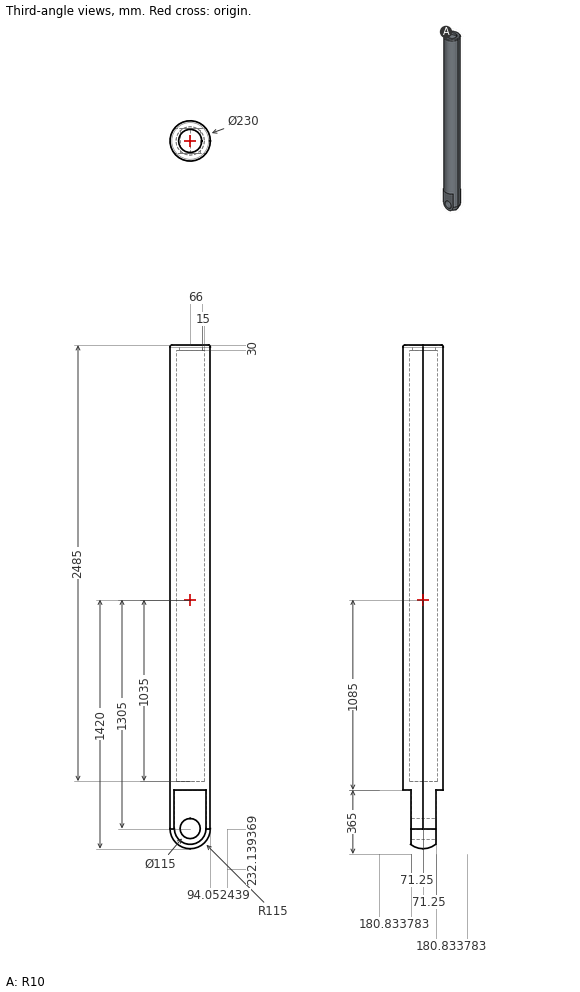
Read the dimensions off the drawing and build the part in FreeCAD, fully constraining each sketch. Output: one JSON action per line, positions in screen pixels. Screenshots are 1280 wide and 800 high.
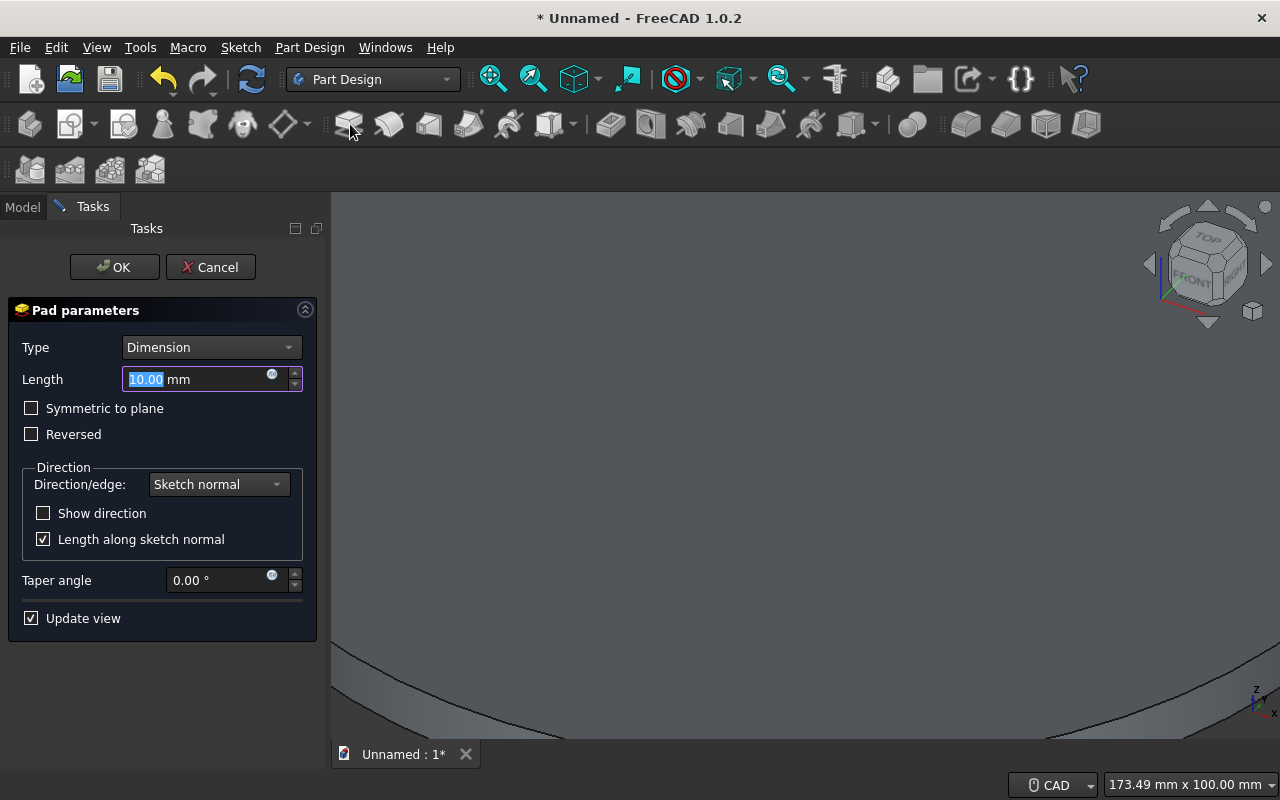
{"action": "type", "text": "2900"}
{"action": "key", "text": "Tab"}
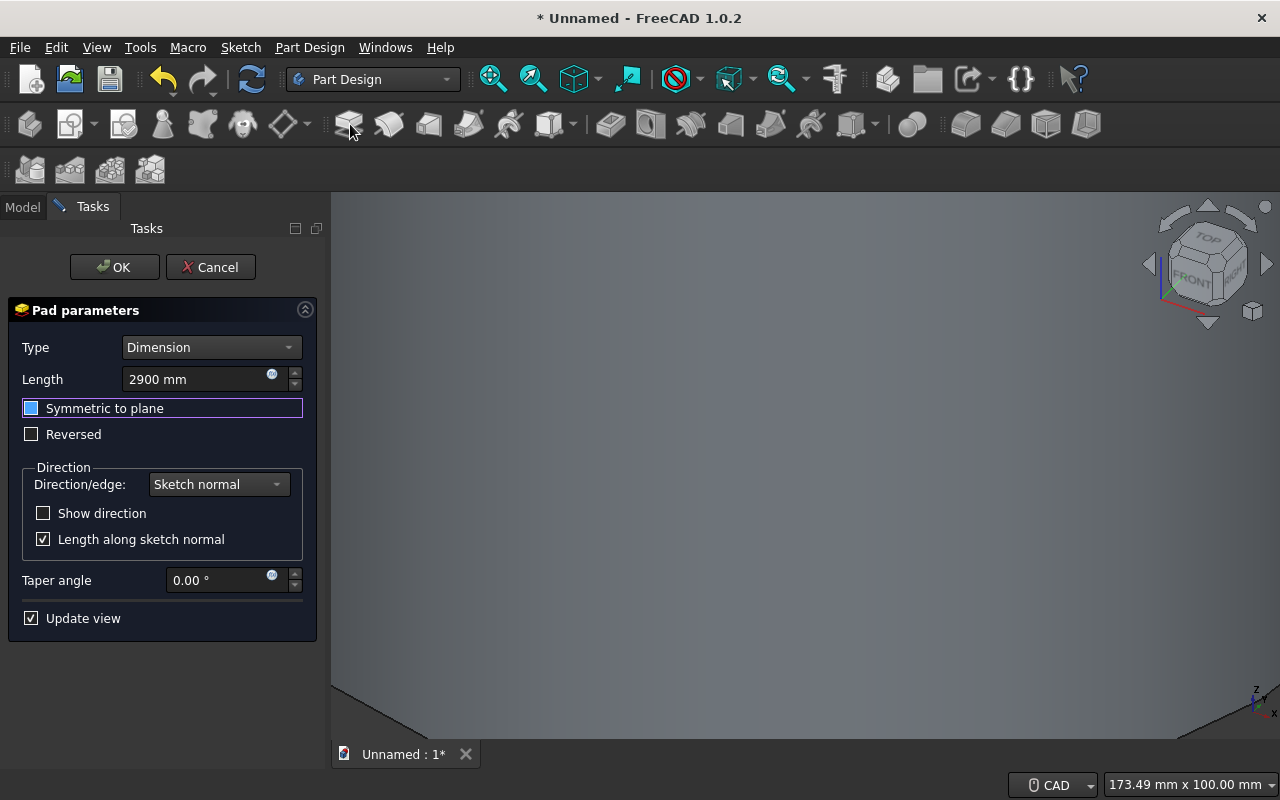
{"action": "left_click", "coordinate": [30, 408]}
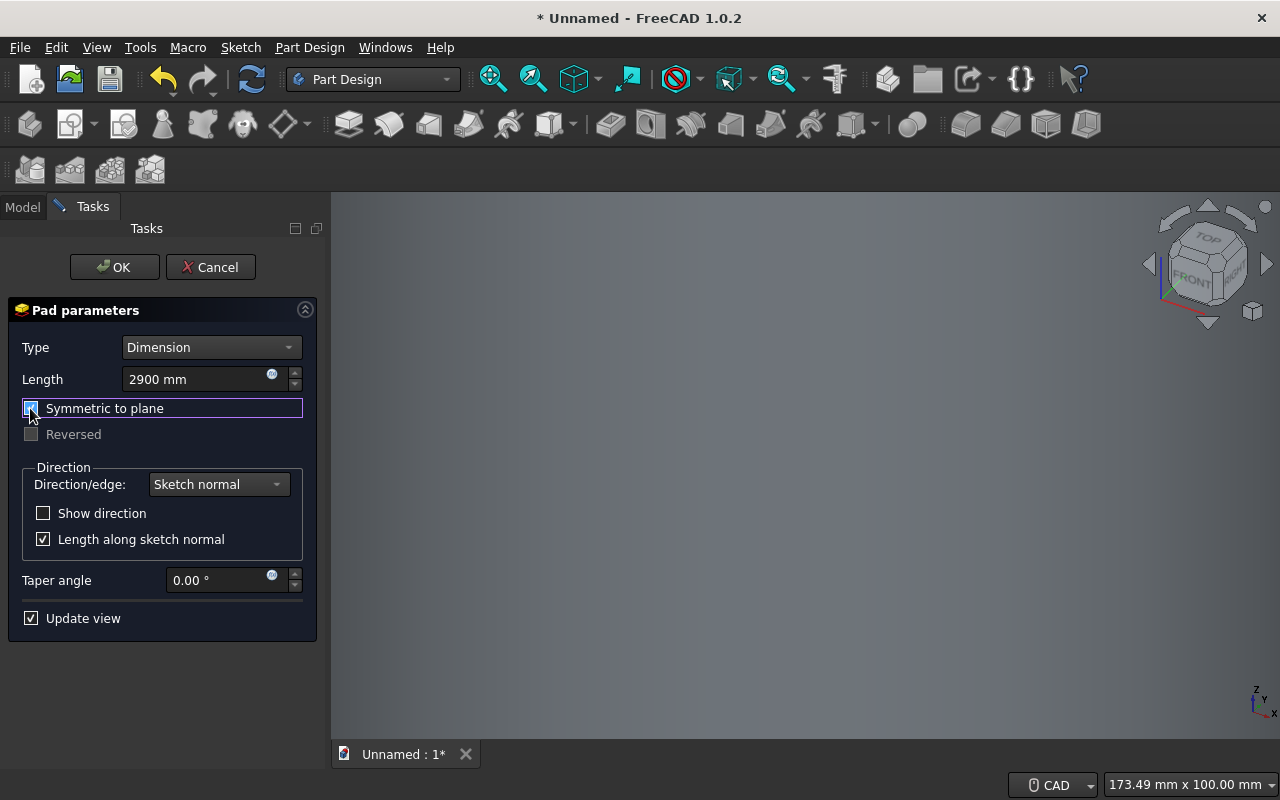
{"action": "left_click", "coordinate": [115, 267]}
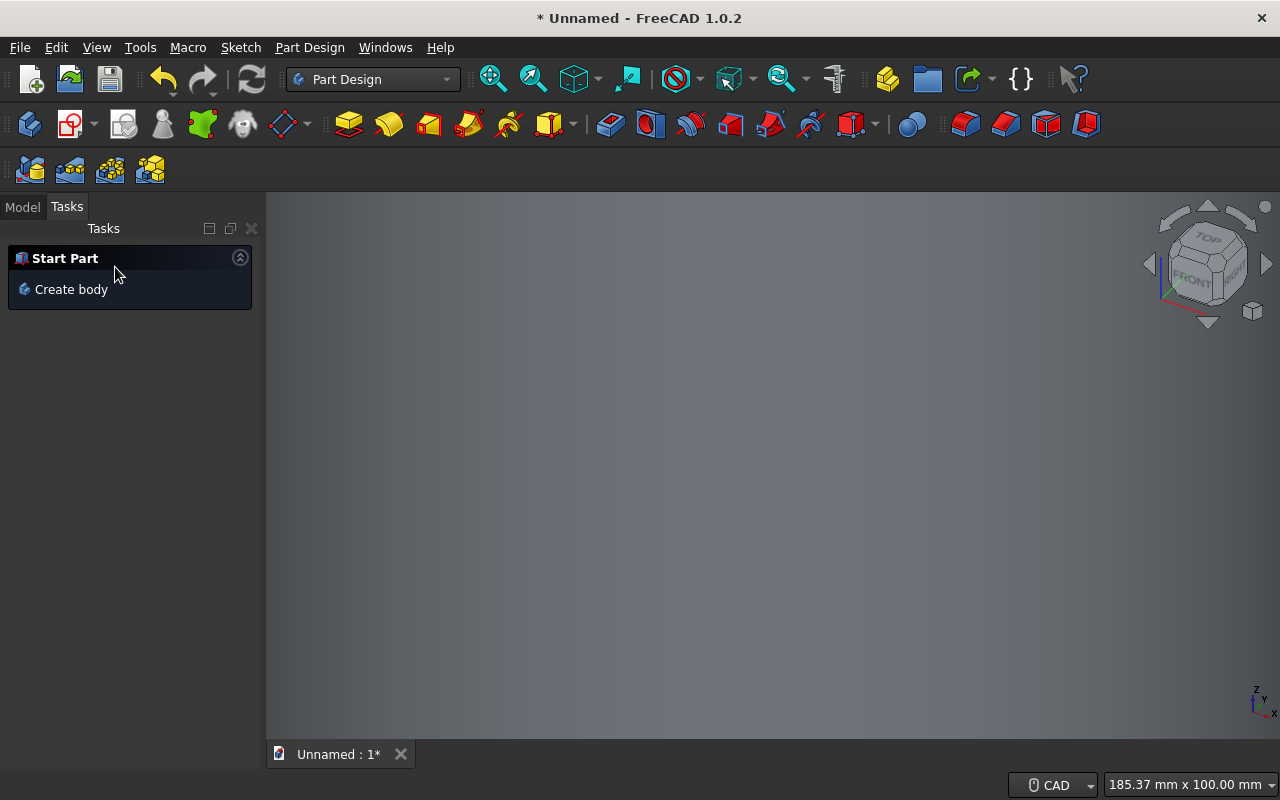
{"action": "key", "text": "v f"}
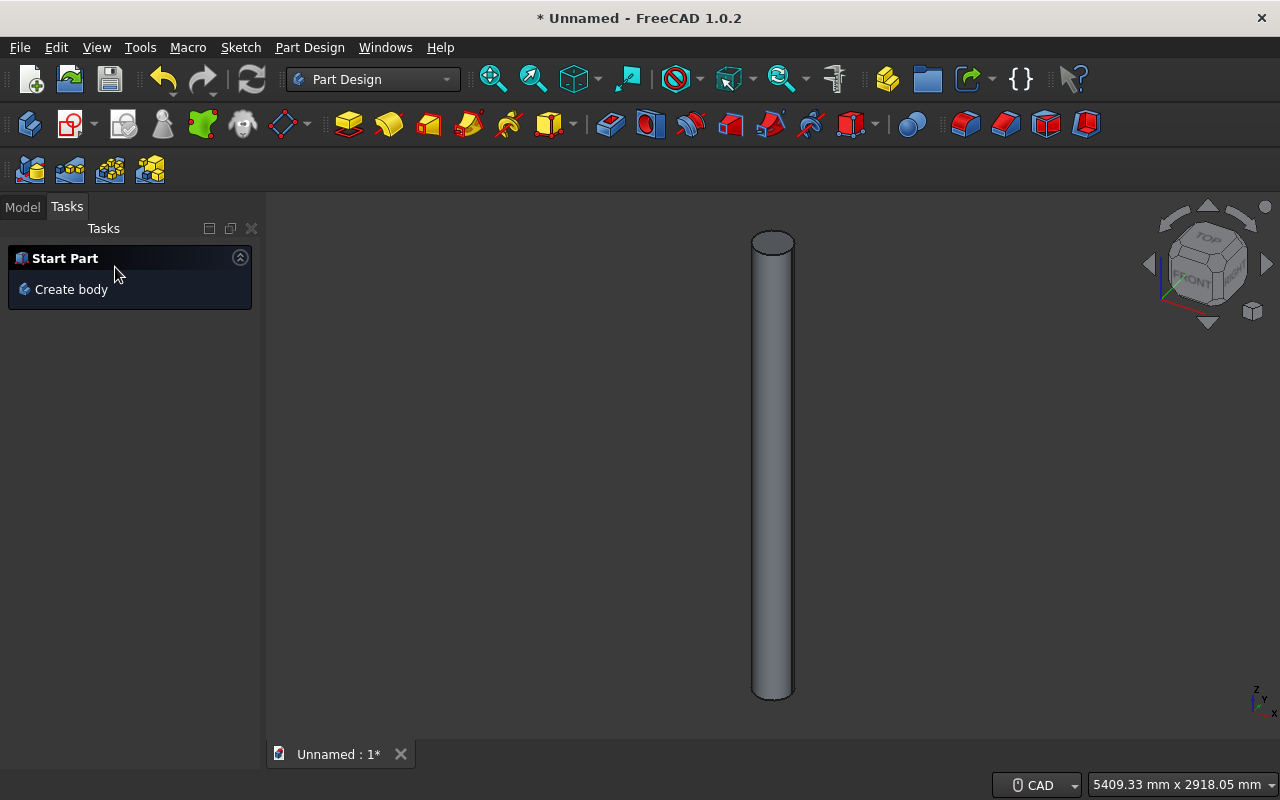
{"action": "left_click", "coordinate": [70, 124]}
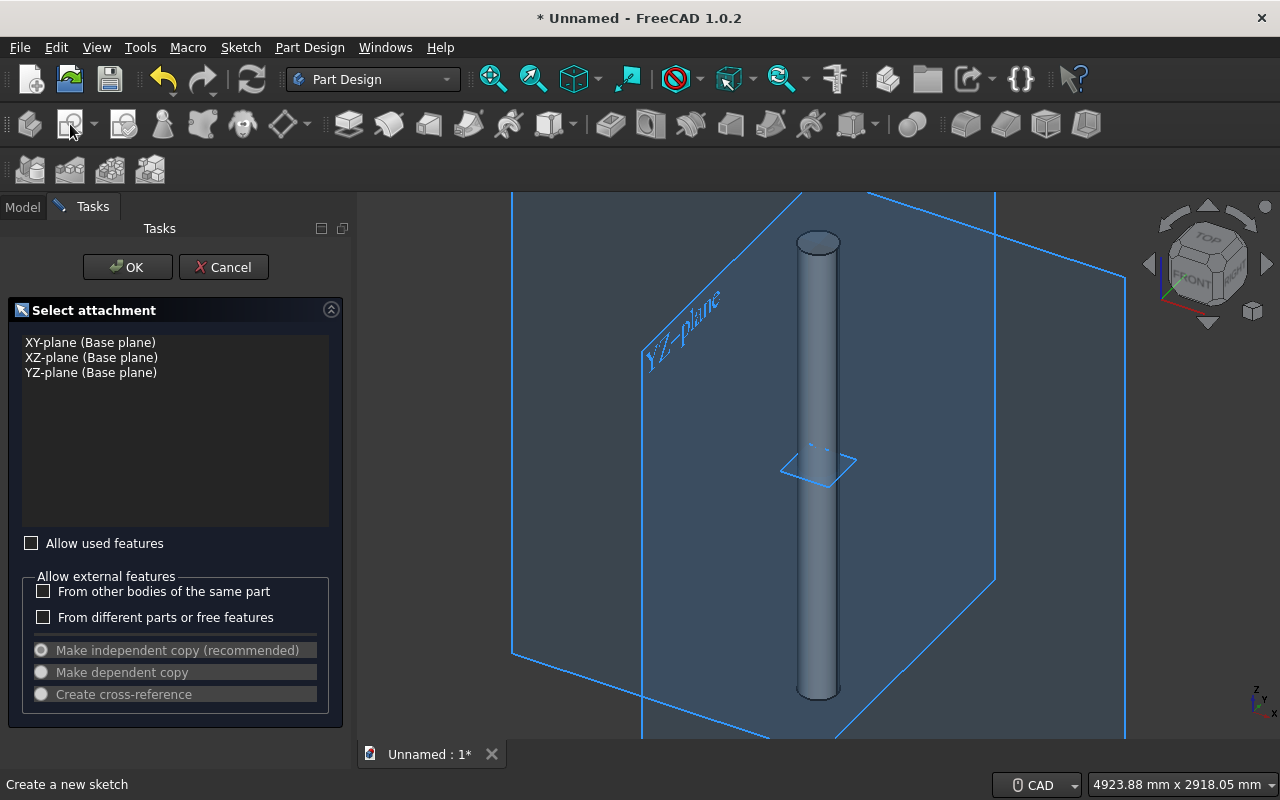
{"action": "left_click", "coordinate": [82, 358]}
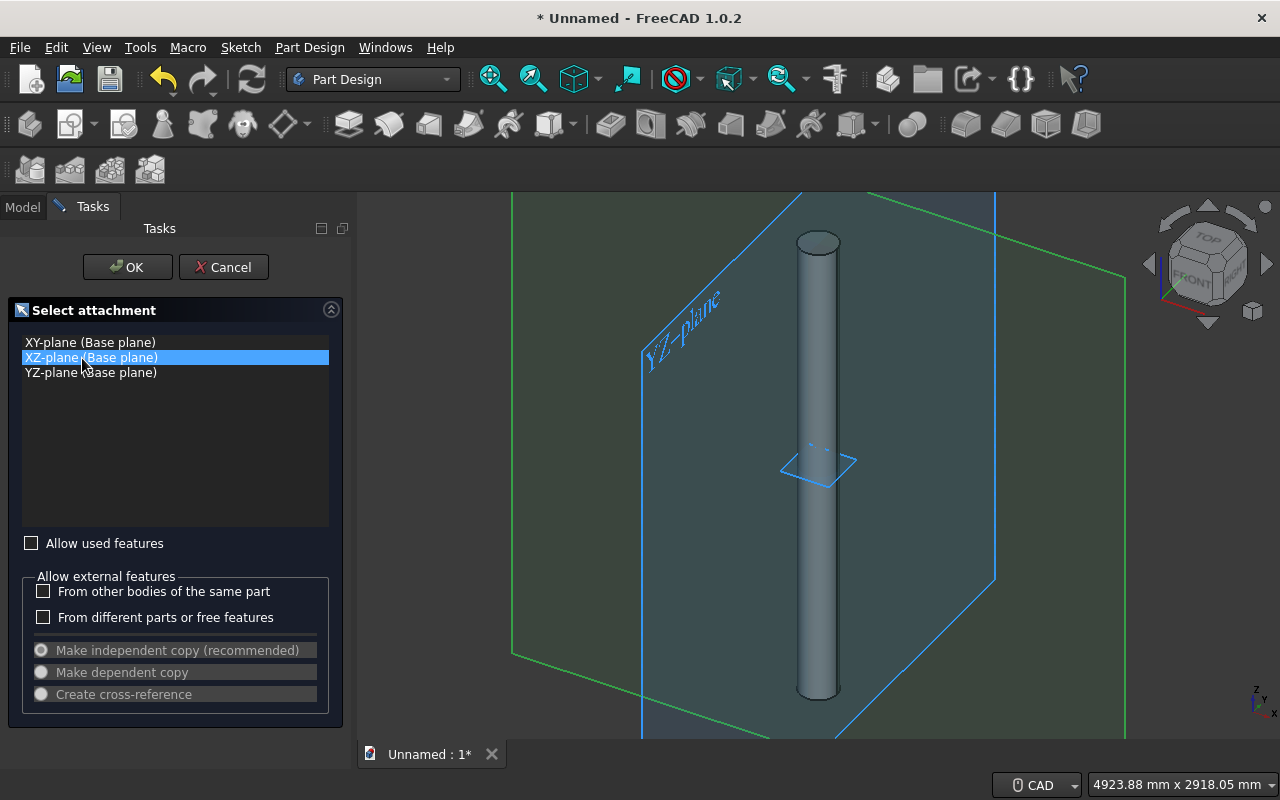
{"action": "left_click", "coordinate": [128, 267]}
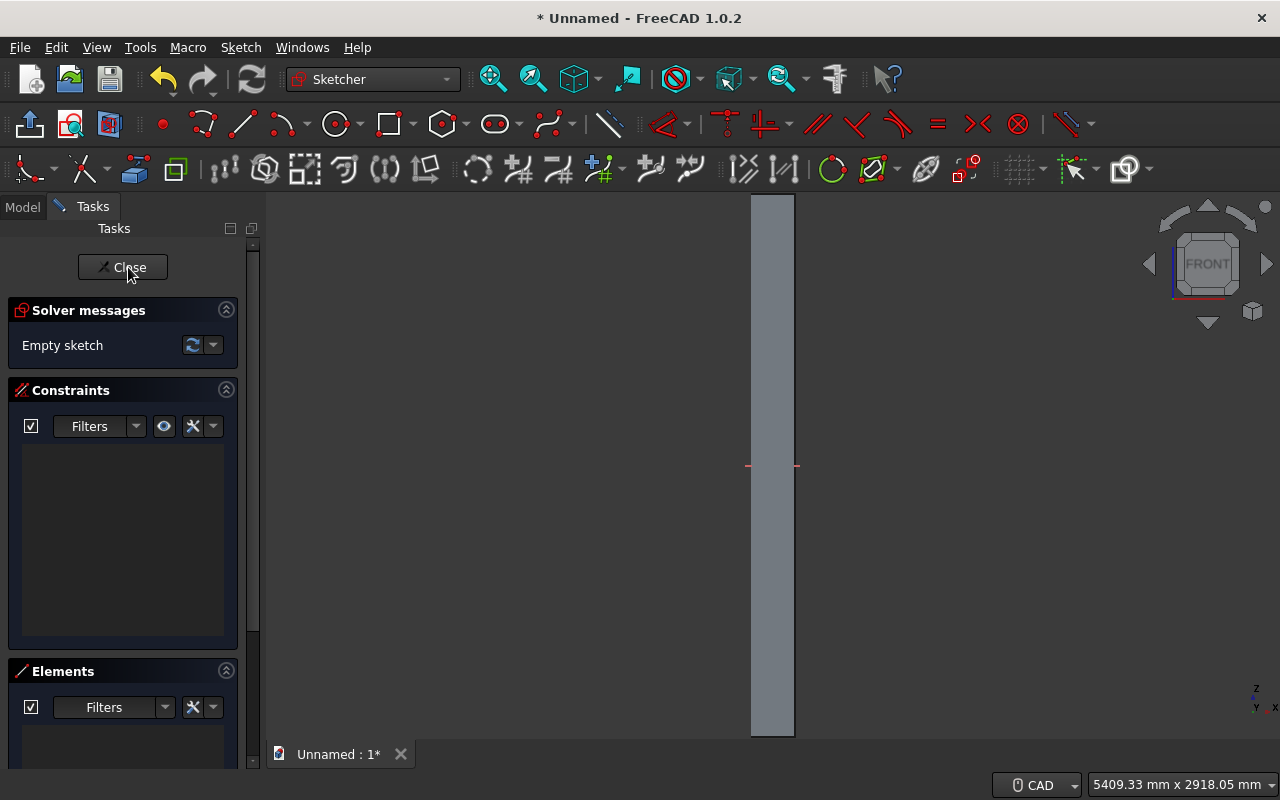
{"action": "key", "text": "q s"}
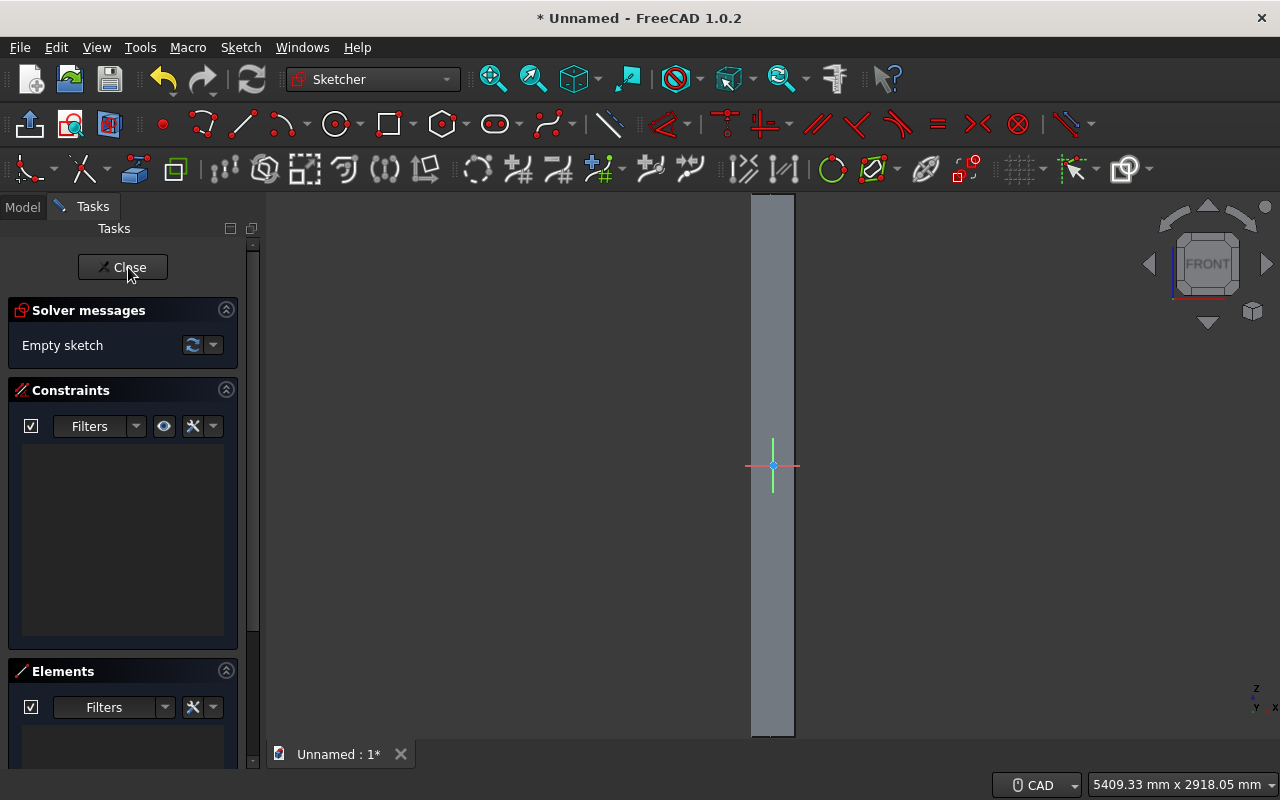
{"action": "scroll", "coordinate": [704, 466], "scroll_direction": "down", "scroll_amount": 5}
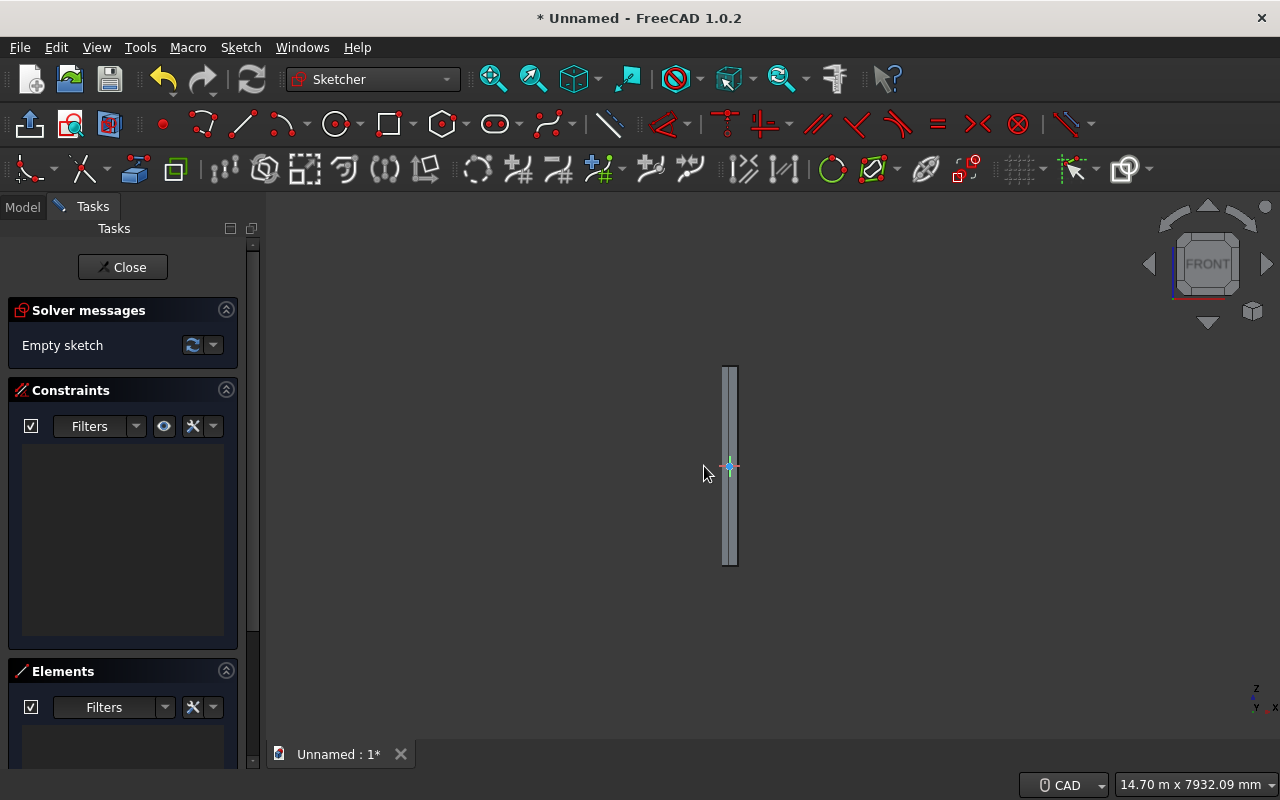
{"action": "scroll", "coordinate": [731, 561], "scroll_direction": "up", "scroll_amount": 15}